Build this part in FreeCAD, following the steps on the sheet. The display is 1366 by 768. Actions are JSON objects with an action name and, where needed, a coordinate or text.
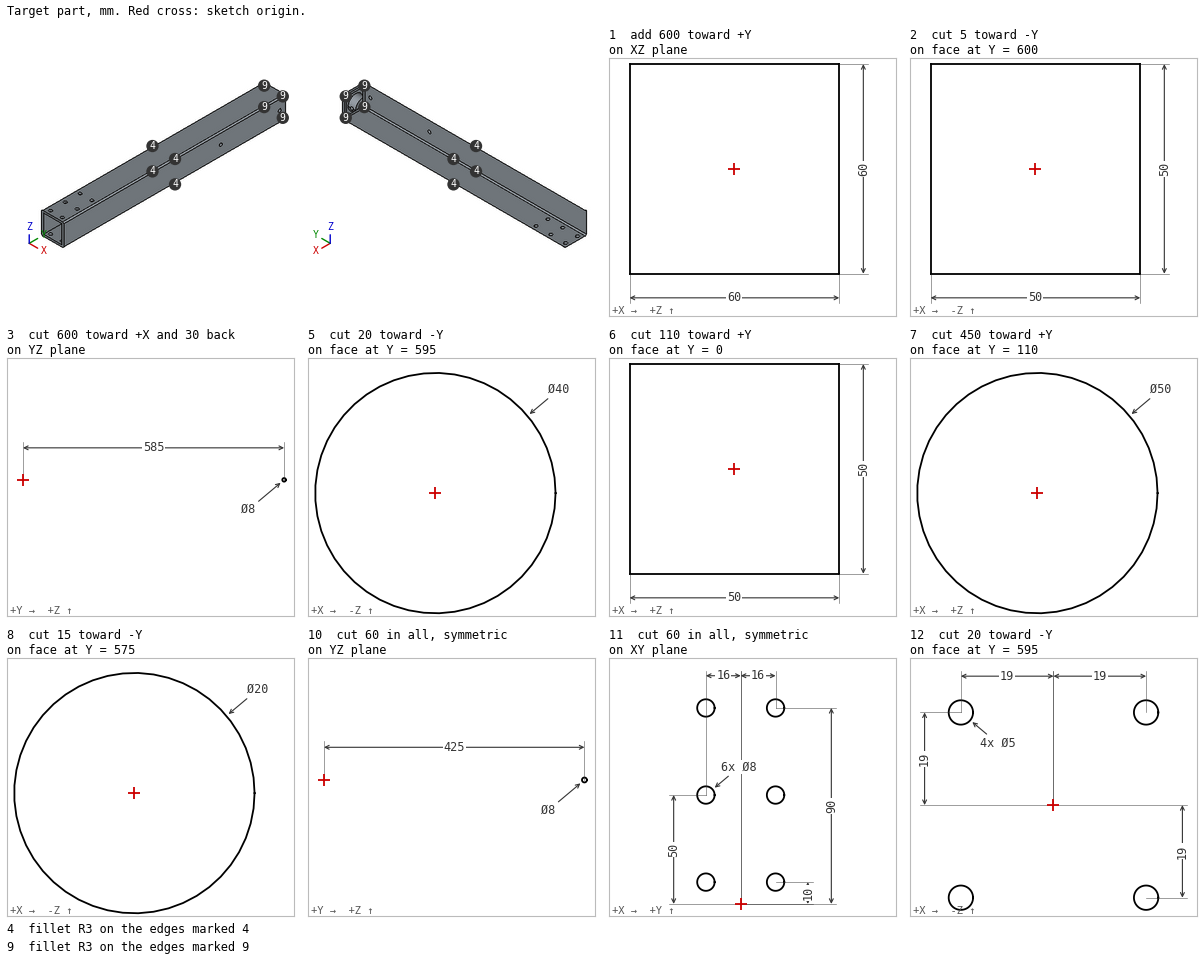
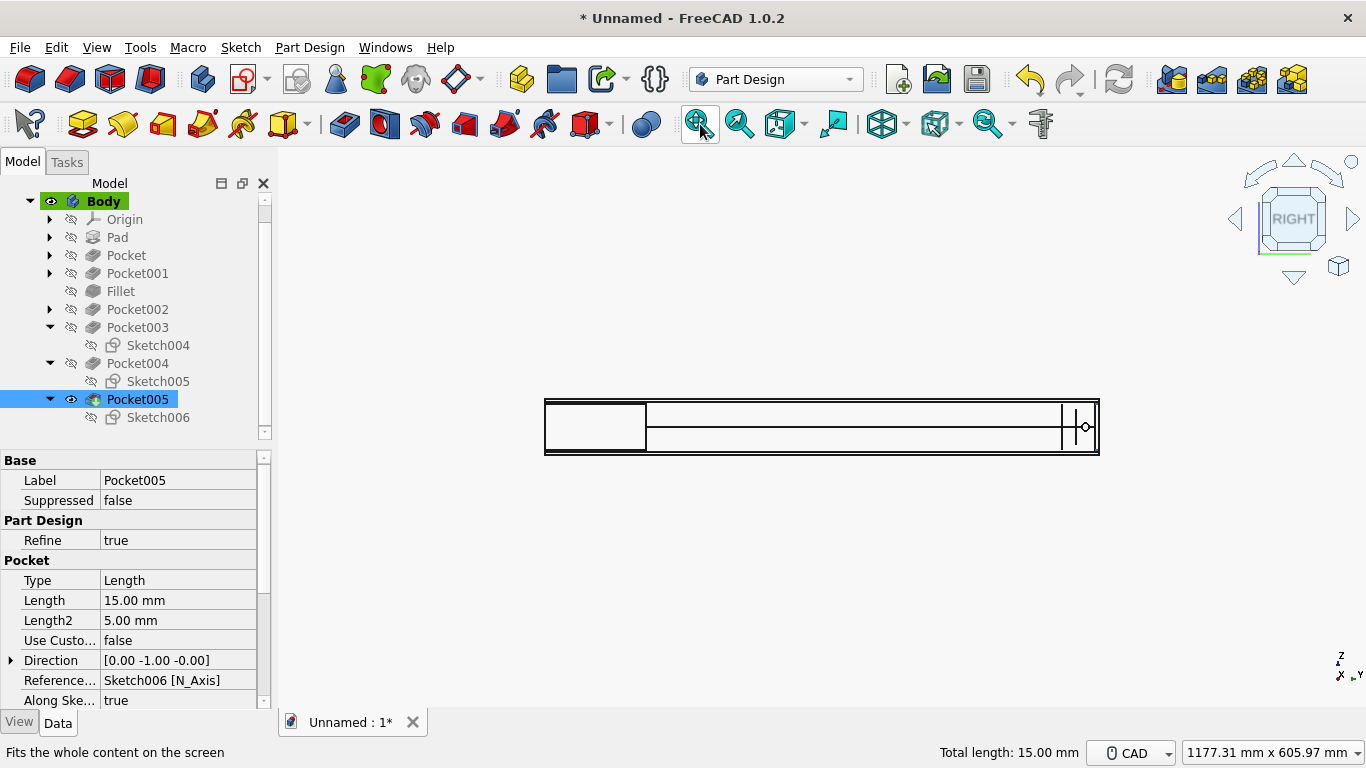
{"action": "key", "text": "5"}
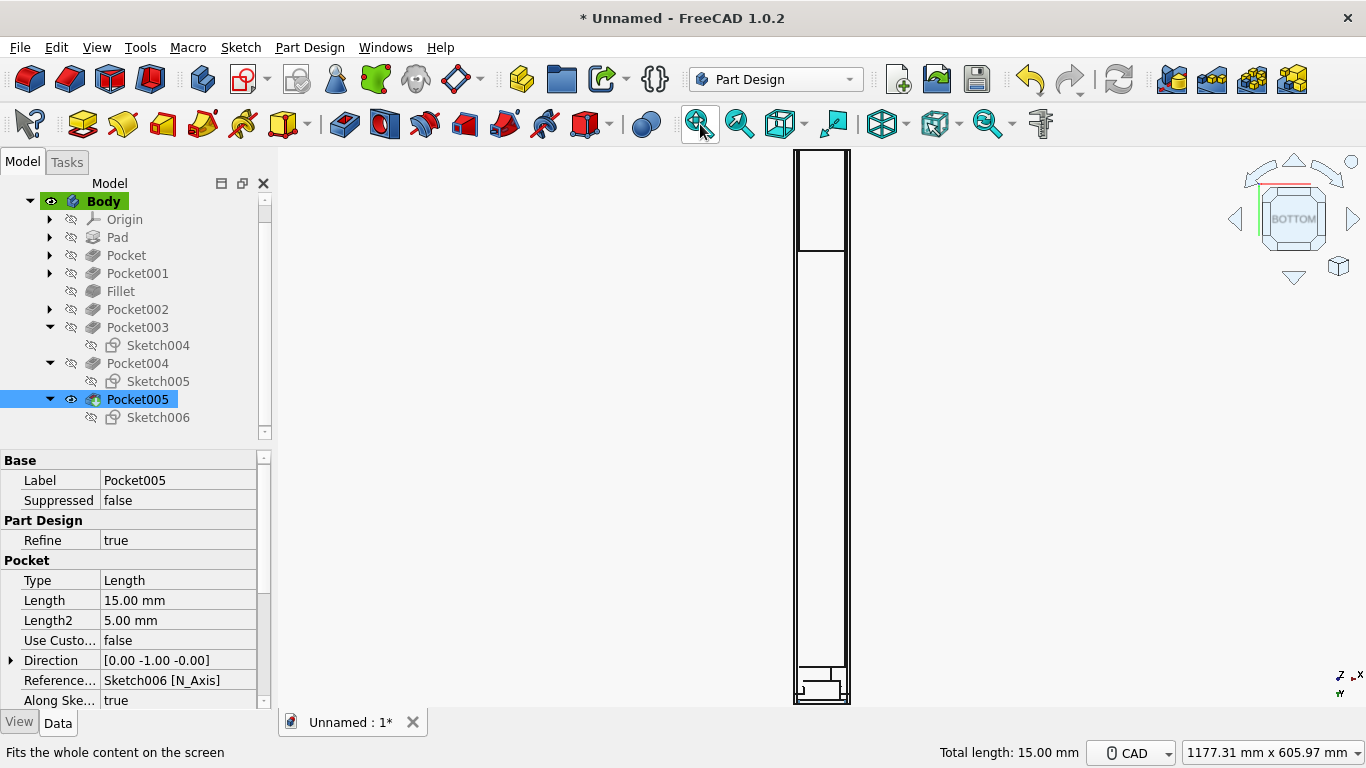
{"action": "key", "text": "4"}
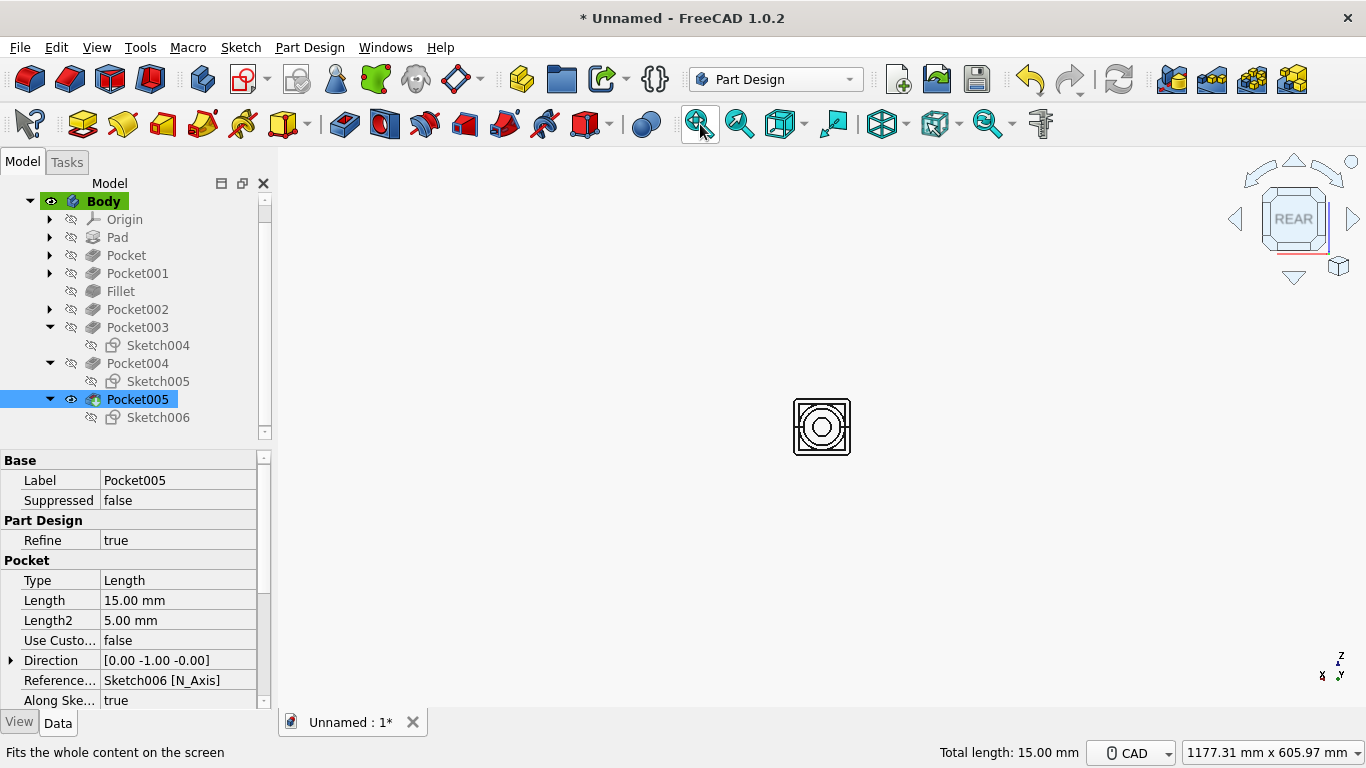
{"action": "left_click", "coordinate": [700, 124]}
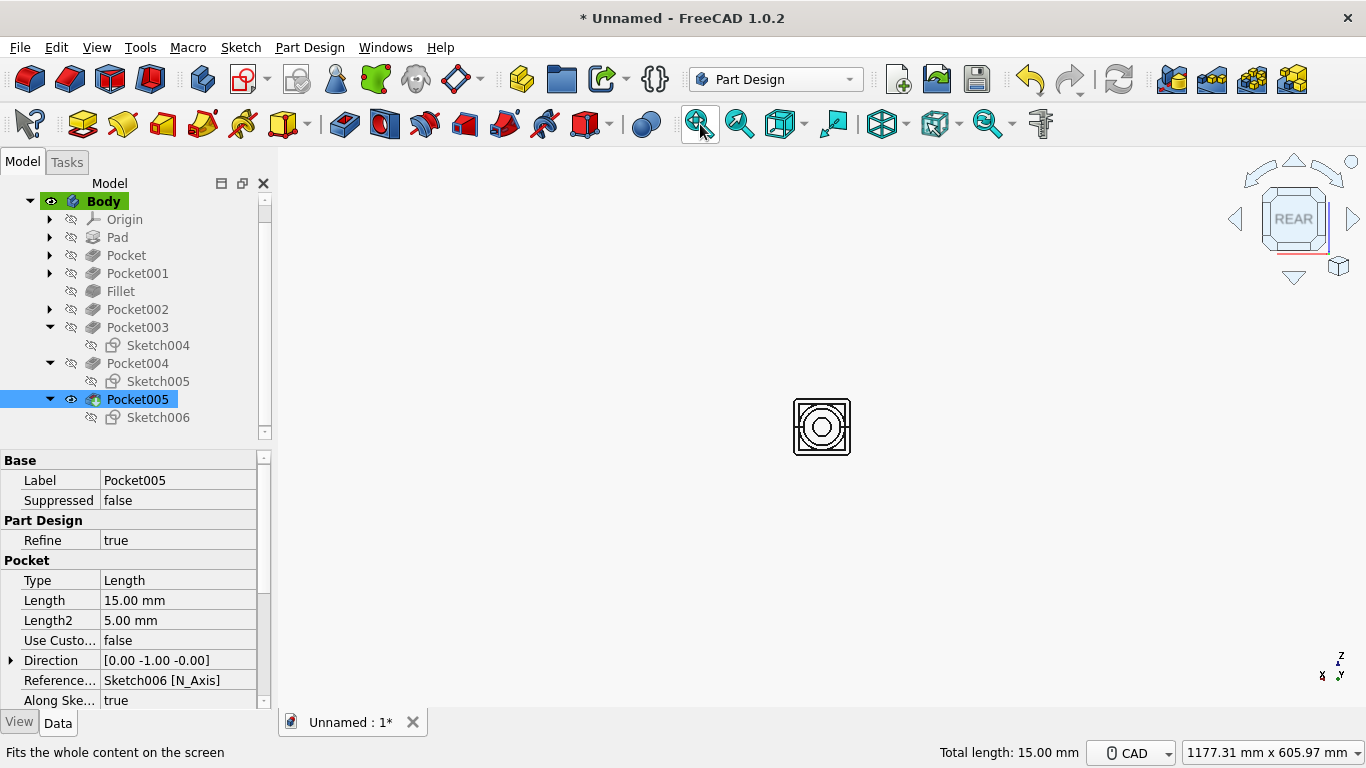
{"action": "scroll", "coordinate": [845, 403], "scroll_direction": "up", "scroll_amount": 11}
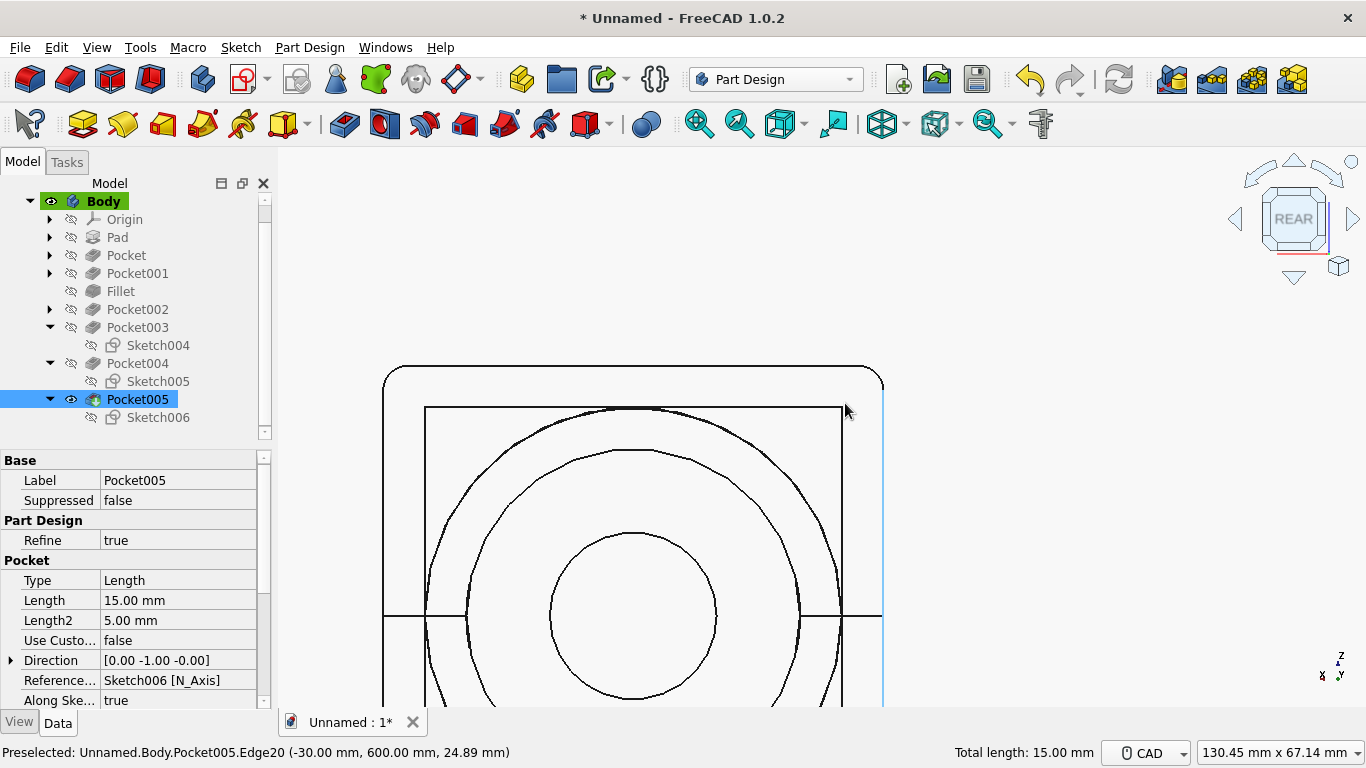
{"action": "left_click", "coordinate": [700, 124]}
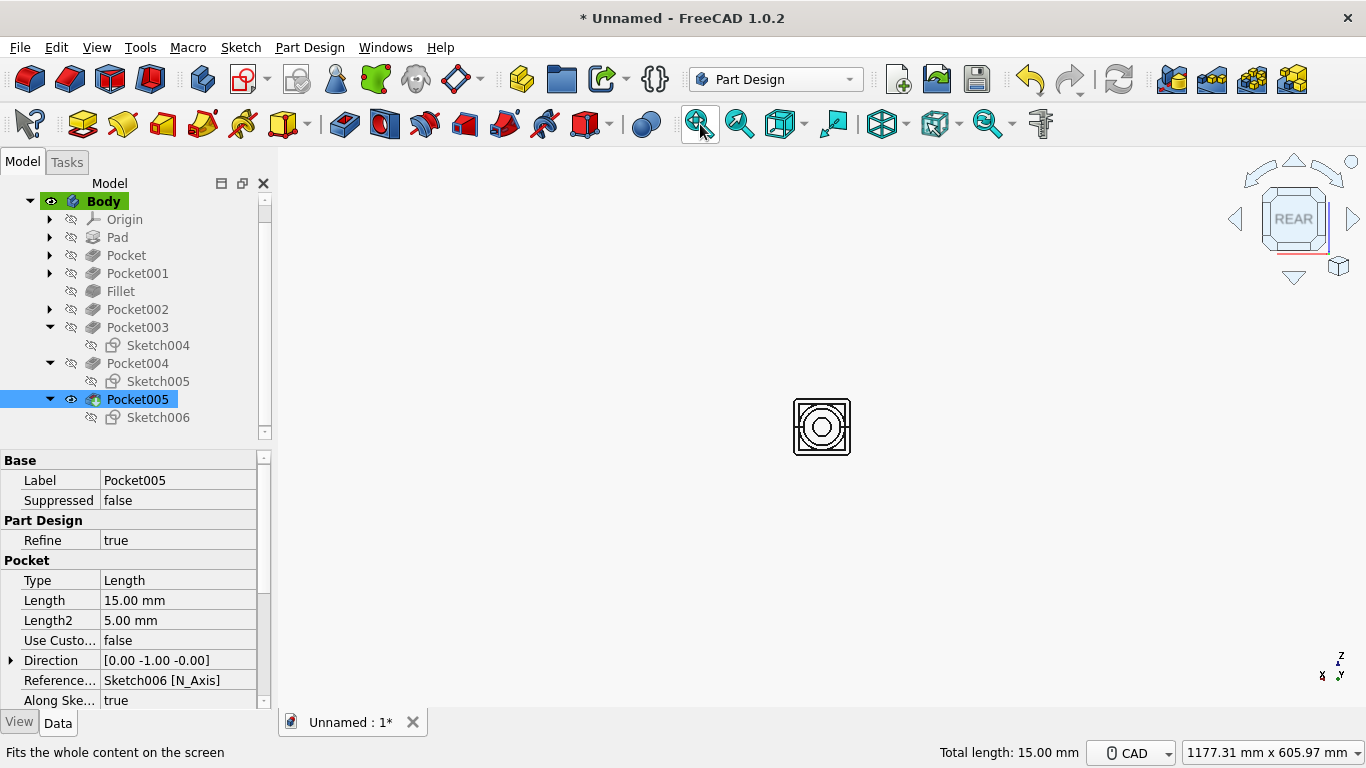
{"action": "key", "text": "6"}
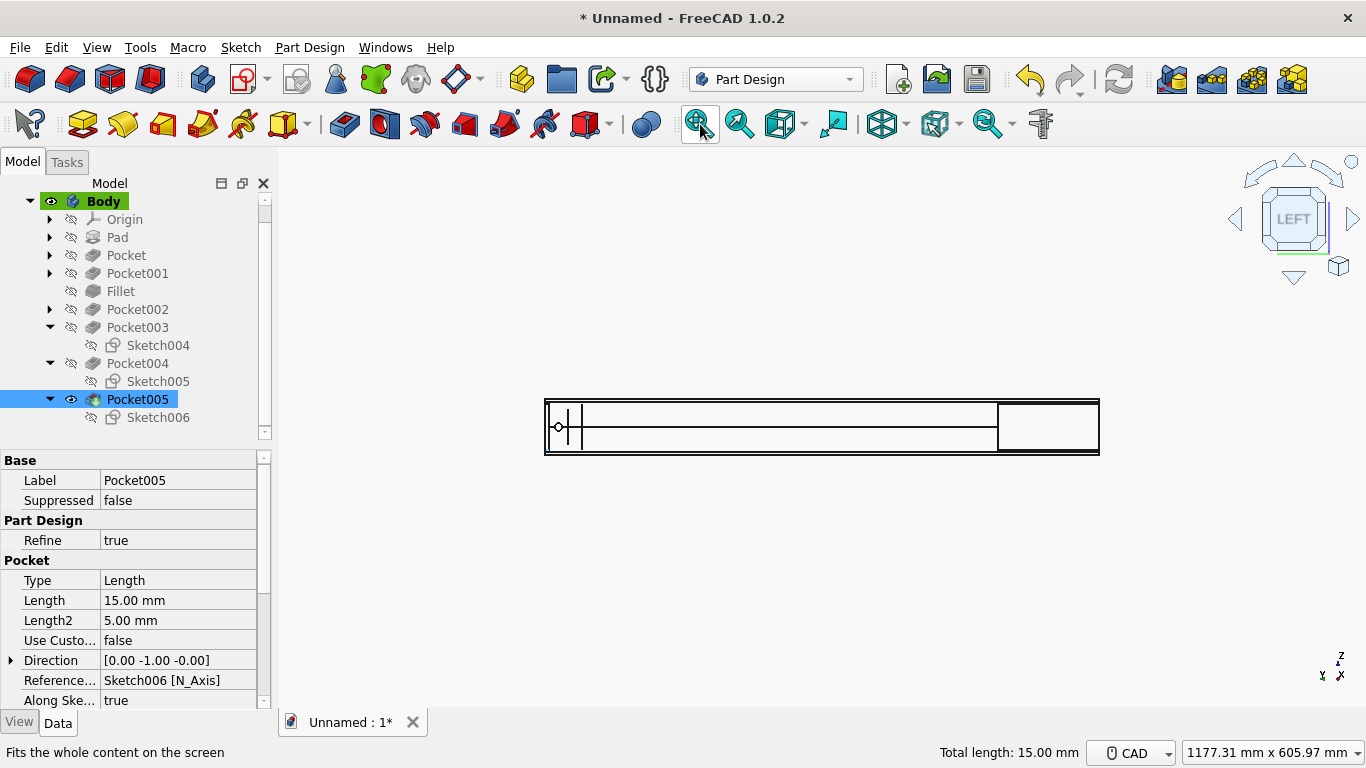
{"action": "scroll", "coordinate": [547, 403], "scroll_direction": "up", "scroll_amount": 11}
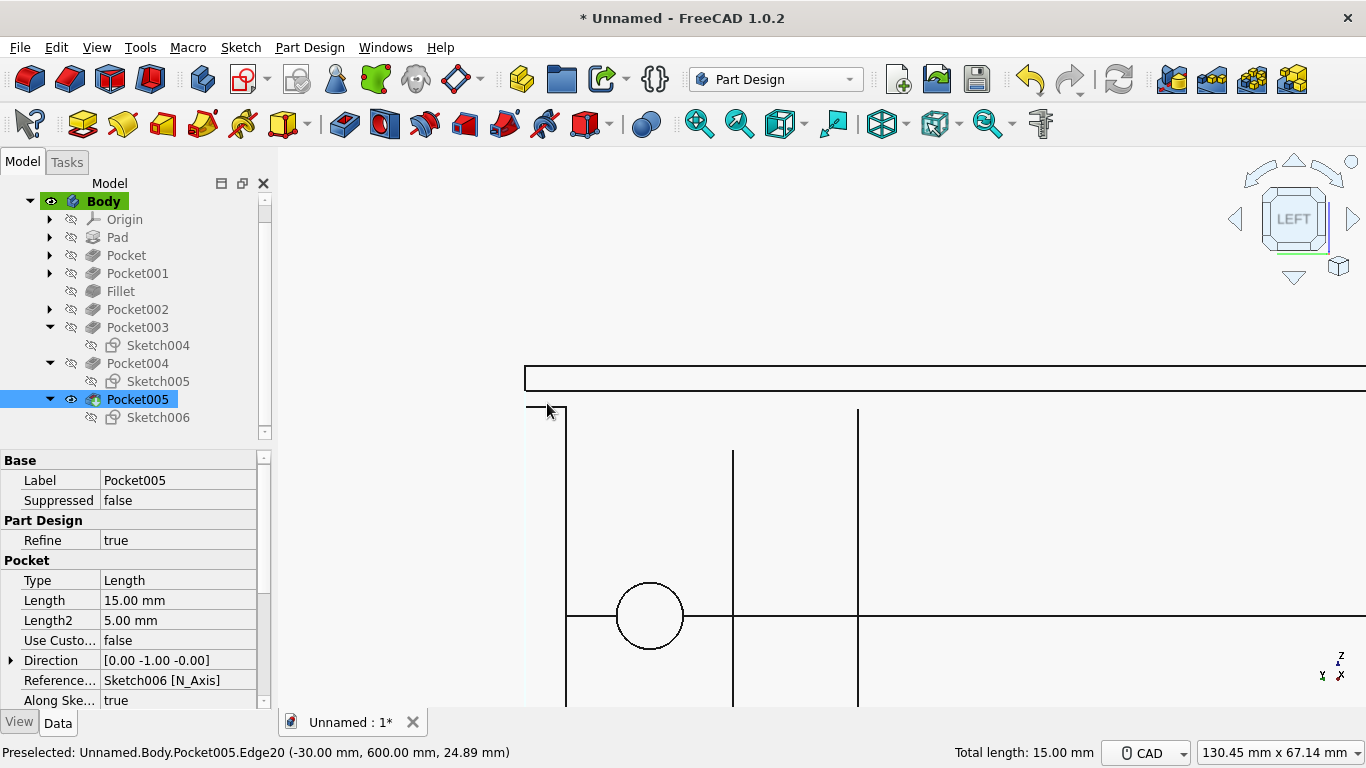
{"action": "left_click", "coordinate": [546, 406], "text": "ctrl"}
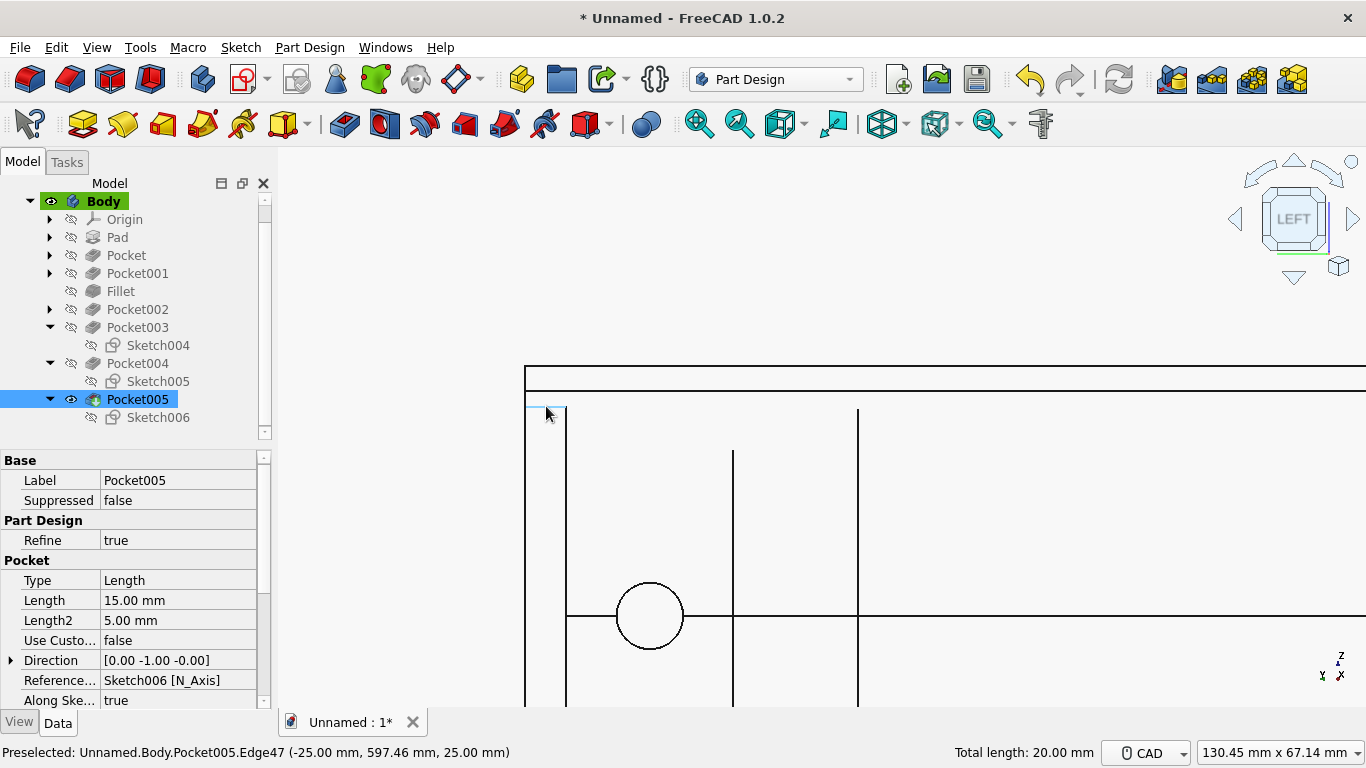
{"action": "key", "text": "v 1"}